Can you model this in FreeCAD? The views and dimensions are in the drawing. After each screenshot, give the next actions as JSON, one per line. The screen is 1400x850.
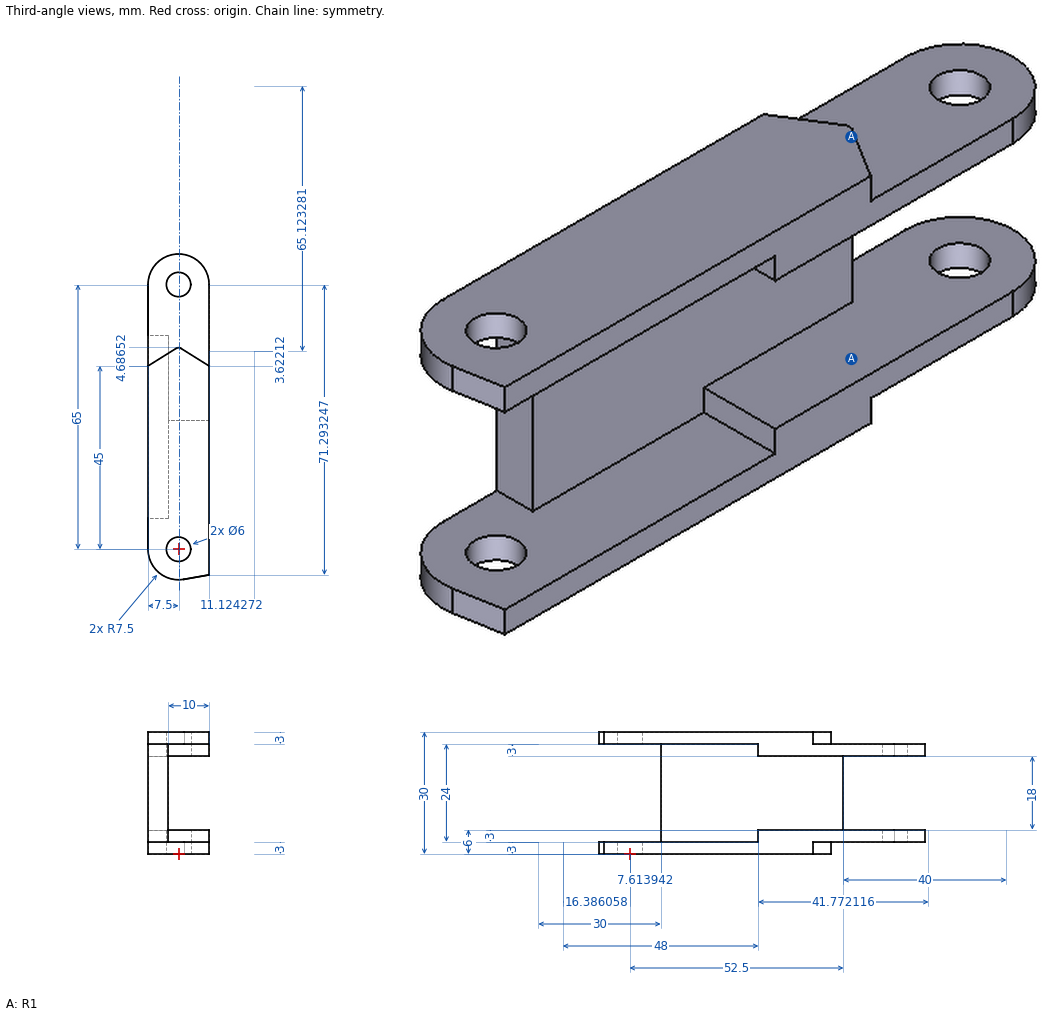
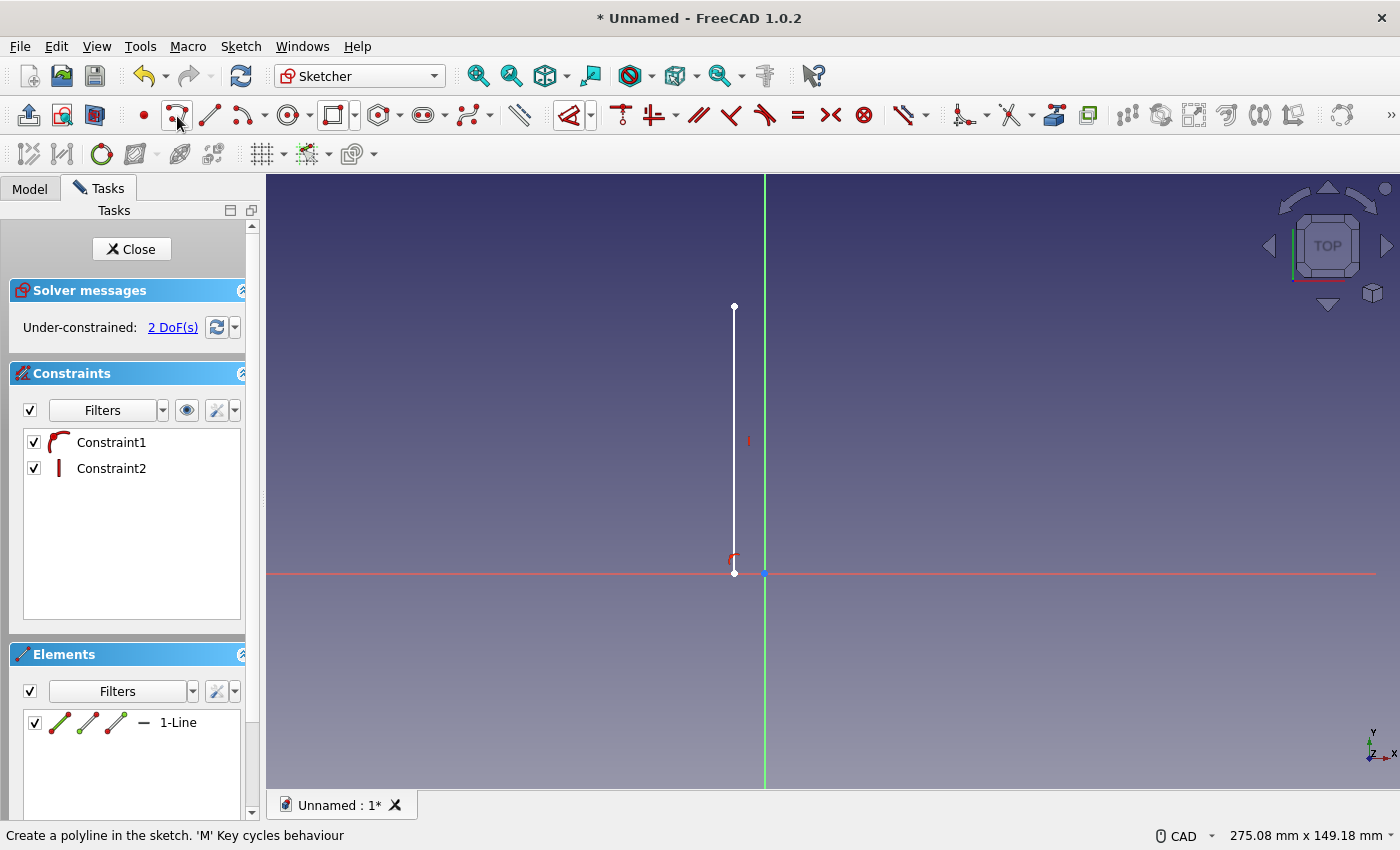
{"action": "scroll", "coordinate": [770, 604], "scroll_direction": "up", "scroll_amount": 6}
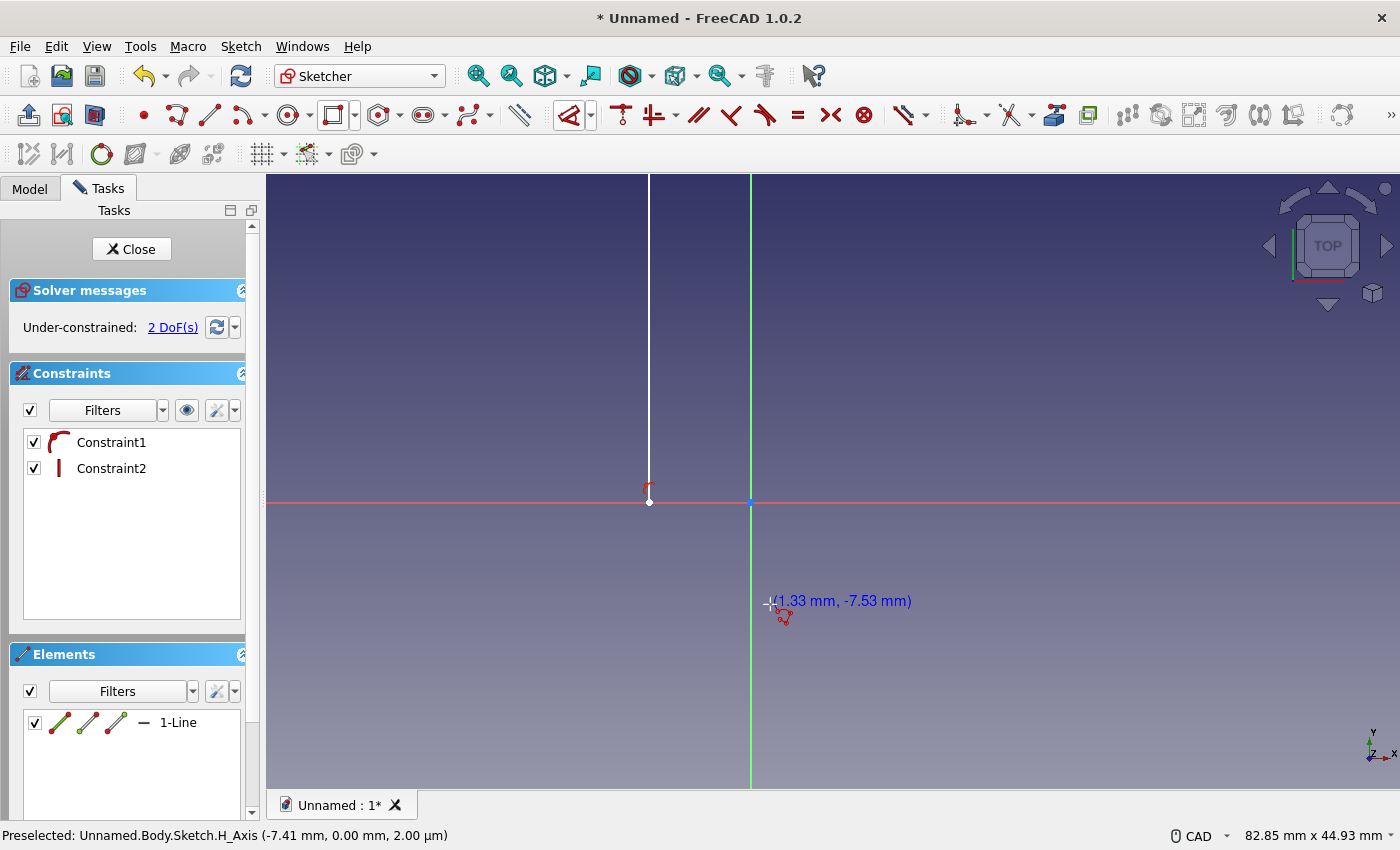
{"action": "left_click", "coordinate": [769, 604]}
{"action": "left_click", "coordinate": [853, 589]}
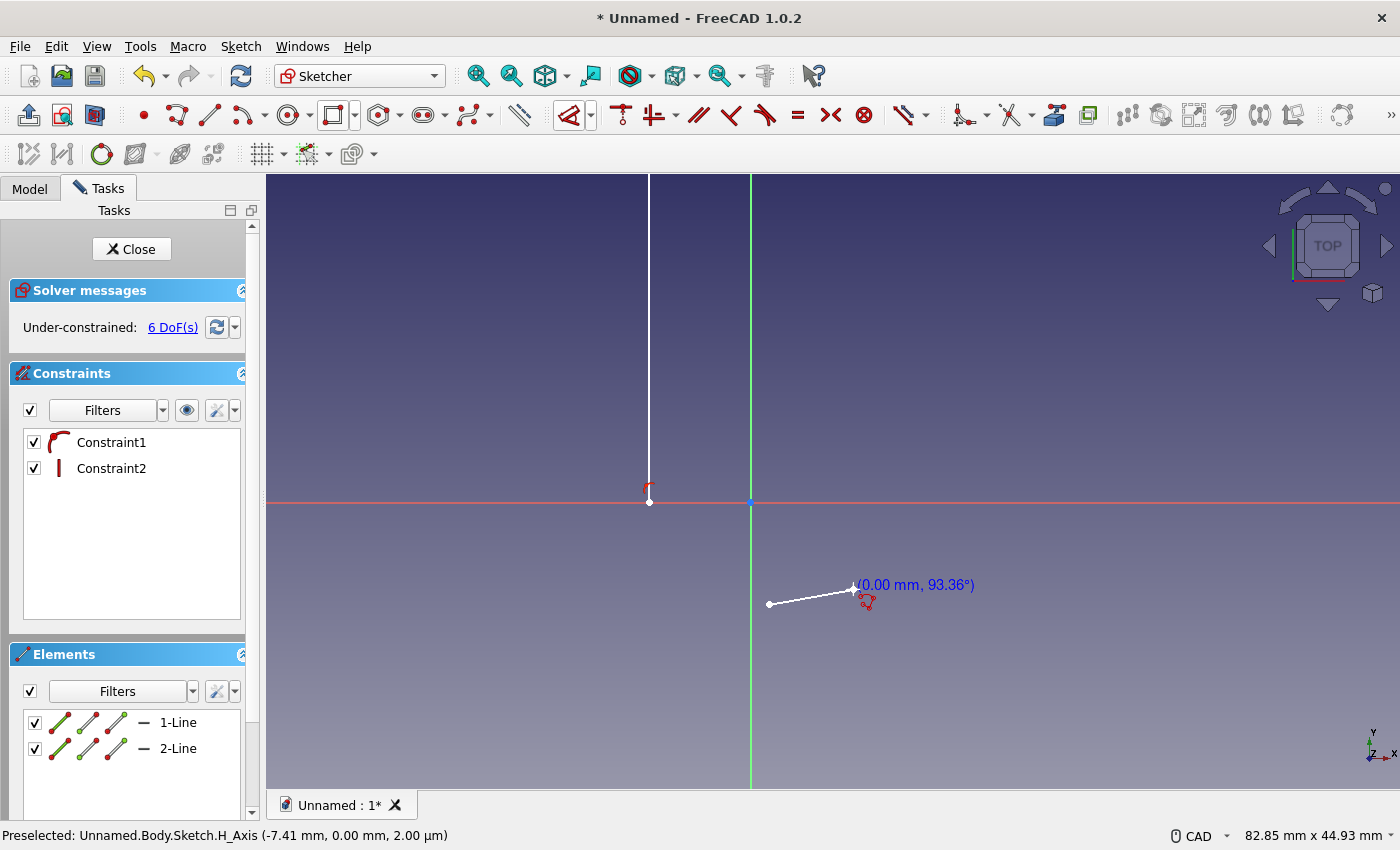
{"action": "scroll", "coordinate": [772, 729], "scroll_direction": "down", "scroll_amount": 5}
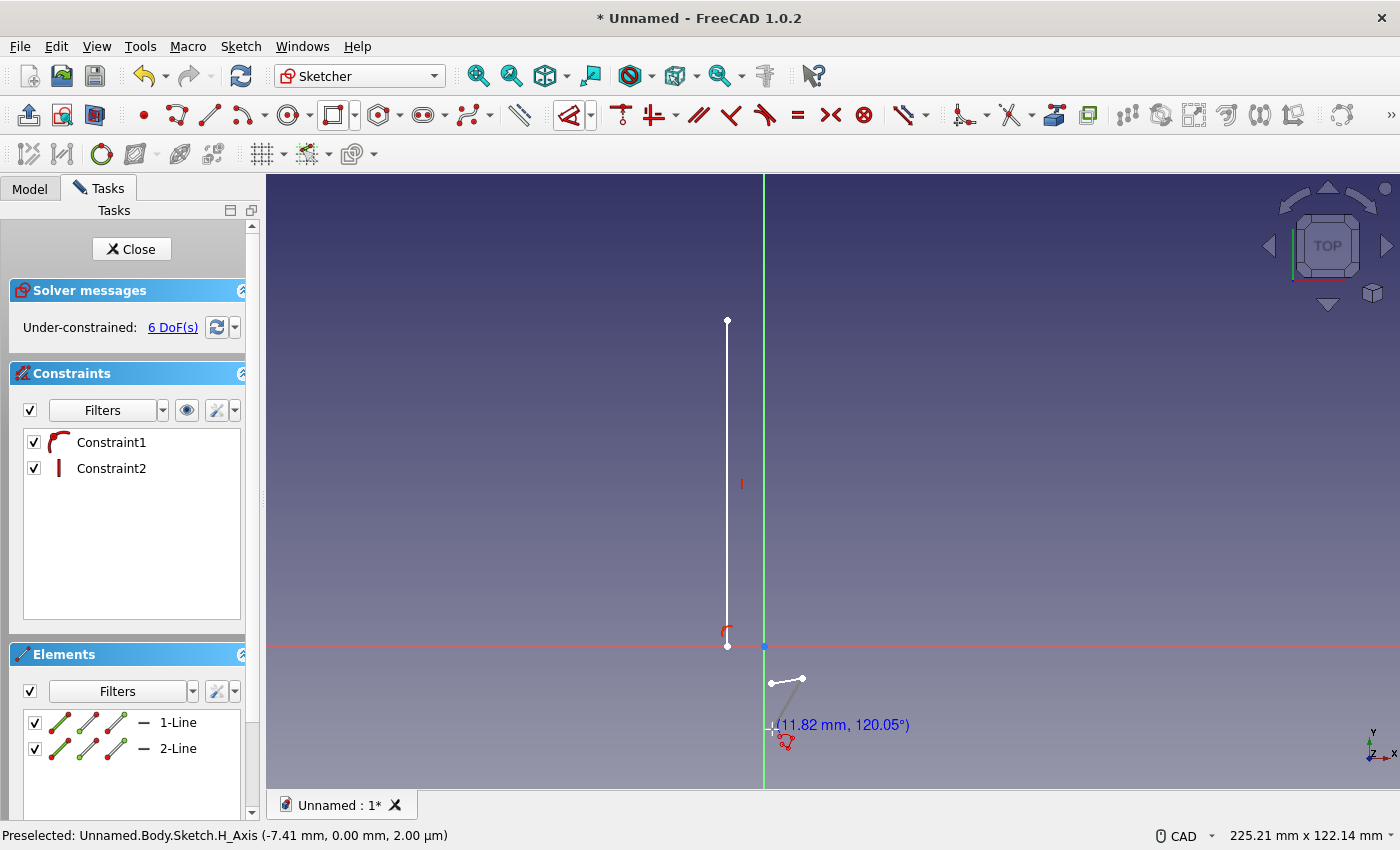
{"action": "left_click", "coordinate": [802, 319]}
{"action": "right_click", "coordinate": [802, 319]}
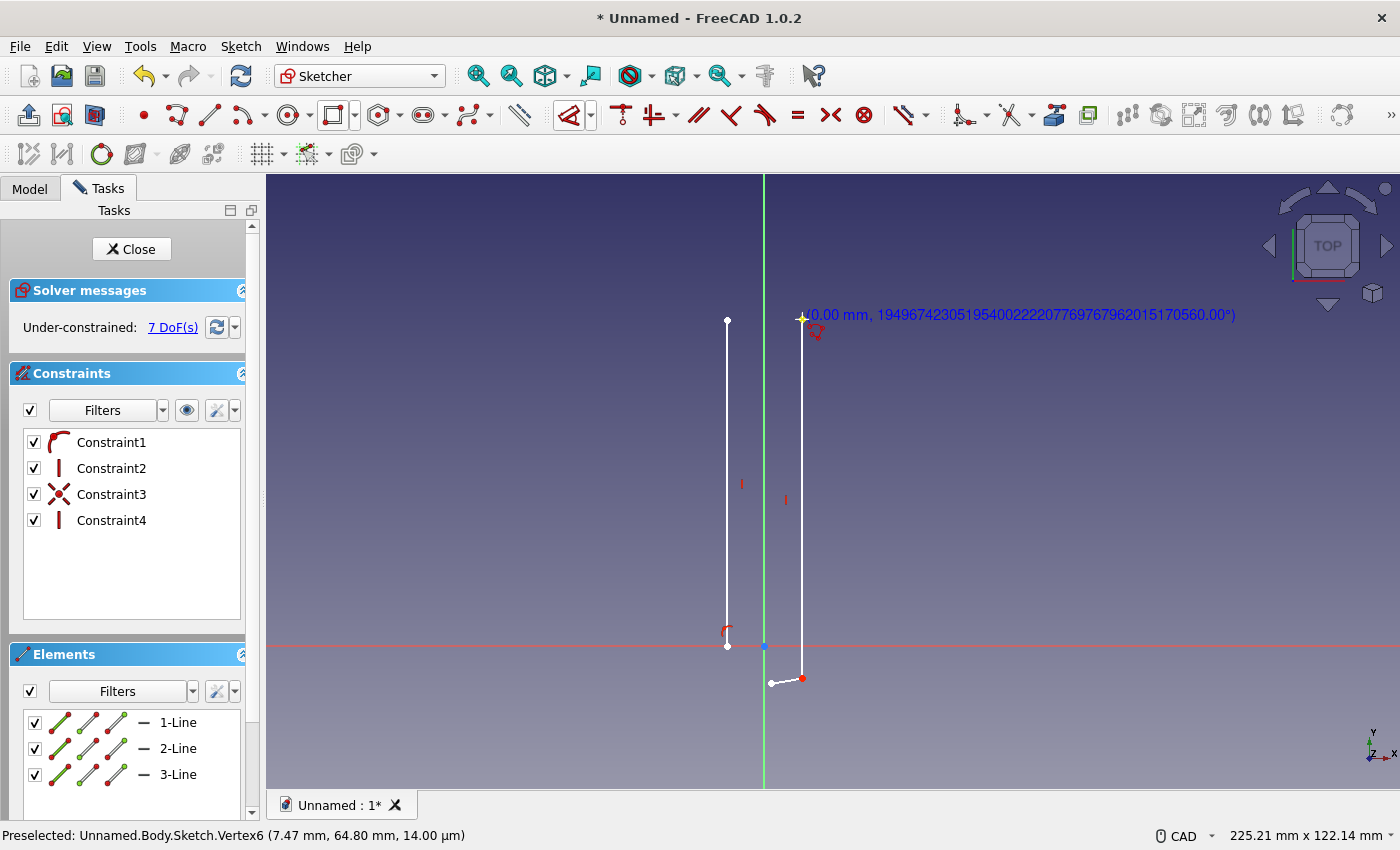
{"action": "key", "text": "g 3 a"}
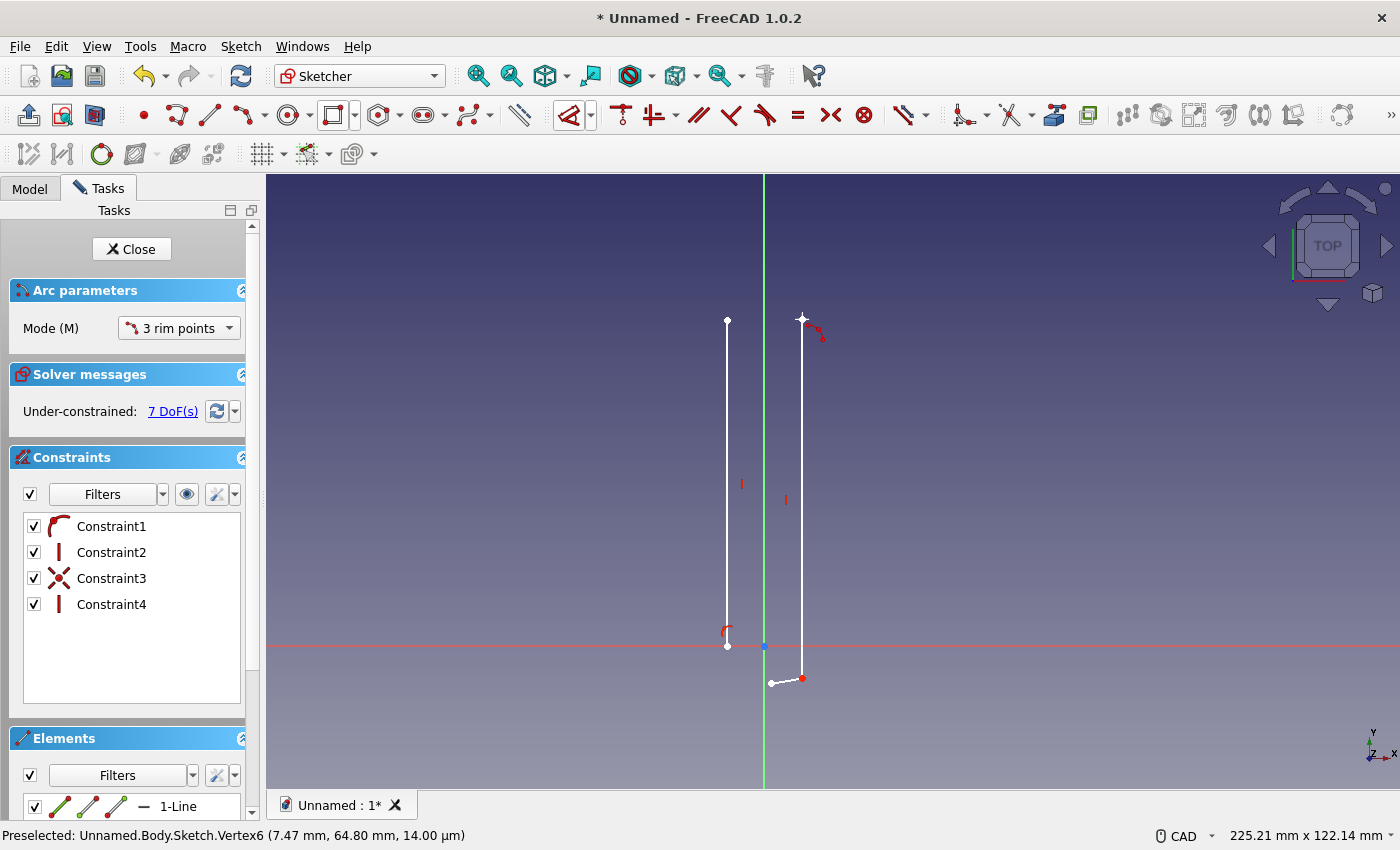
{"action": "left_click", "coordinate": [727, 646]}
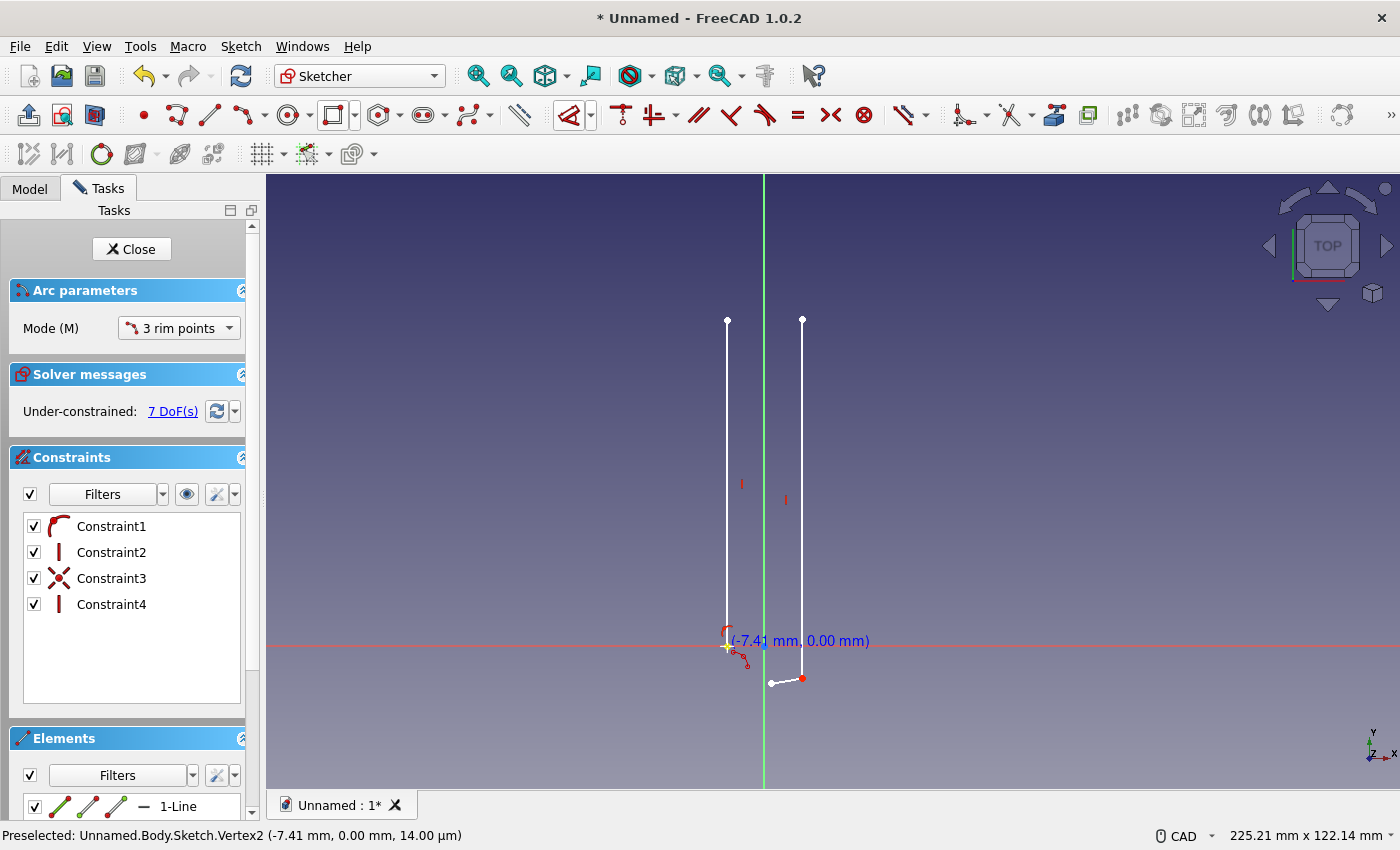
{"action": "scroll", "coordinate": [771, 683], "scroll_direction": "up", "scroll_amount": 5}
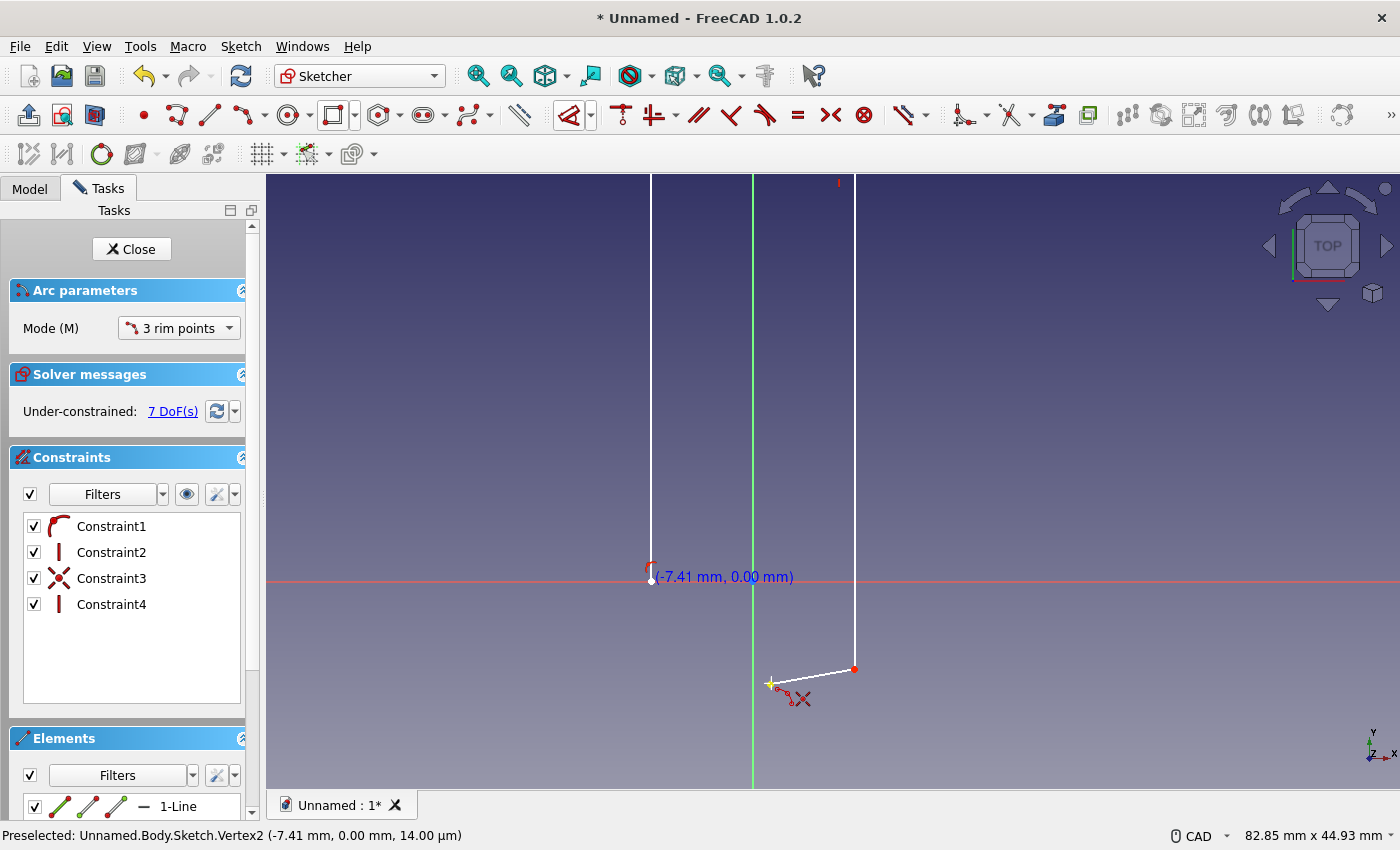
{"action": "left_click", "coordinate": [771, 684]}
{"action": "left_click", "coordinate": [687, 660]}